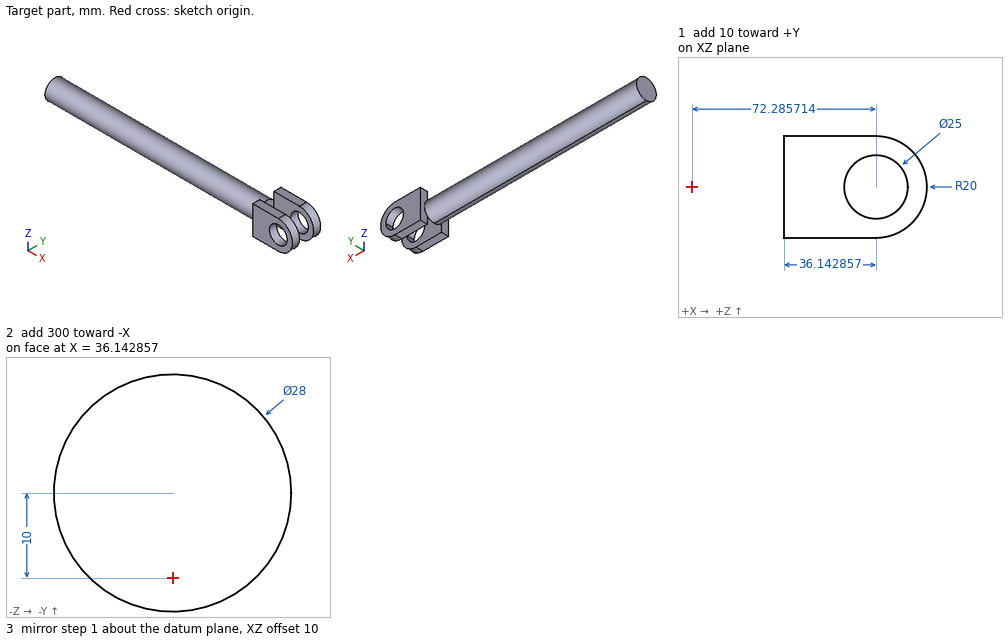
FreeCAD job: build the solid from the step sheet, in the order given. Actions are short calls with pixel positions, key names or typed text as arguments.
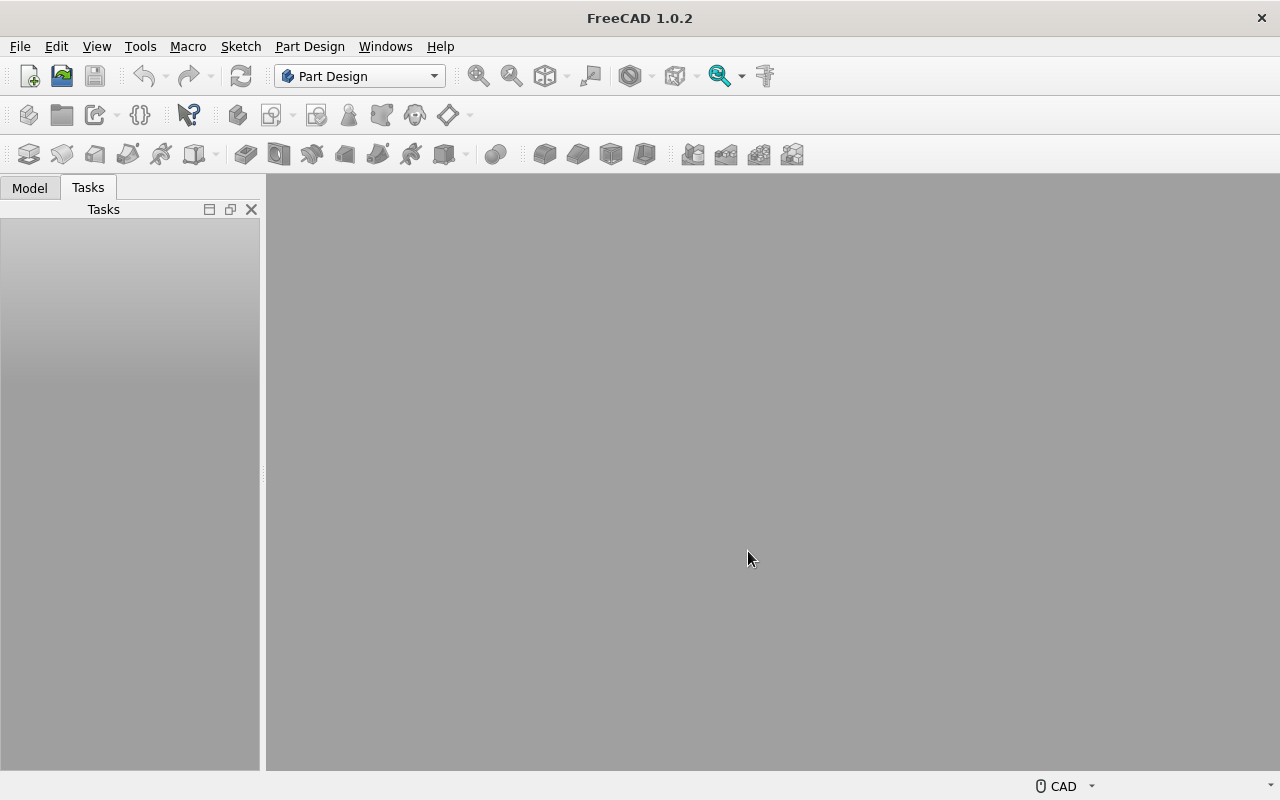
key(ctrl+n)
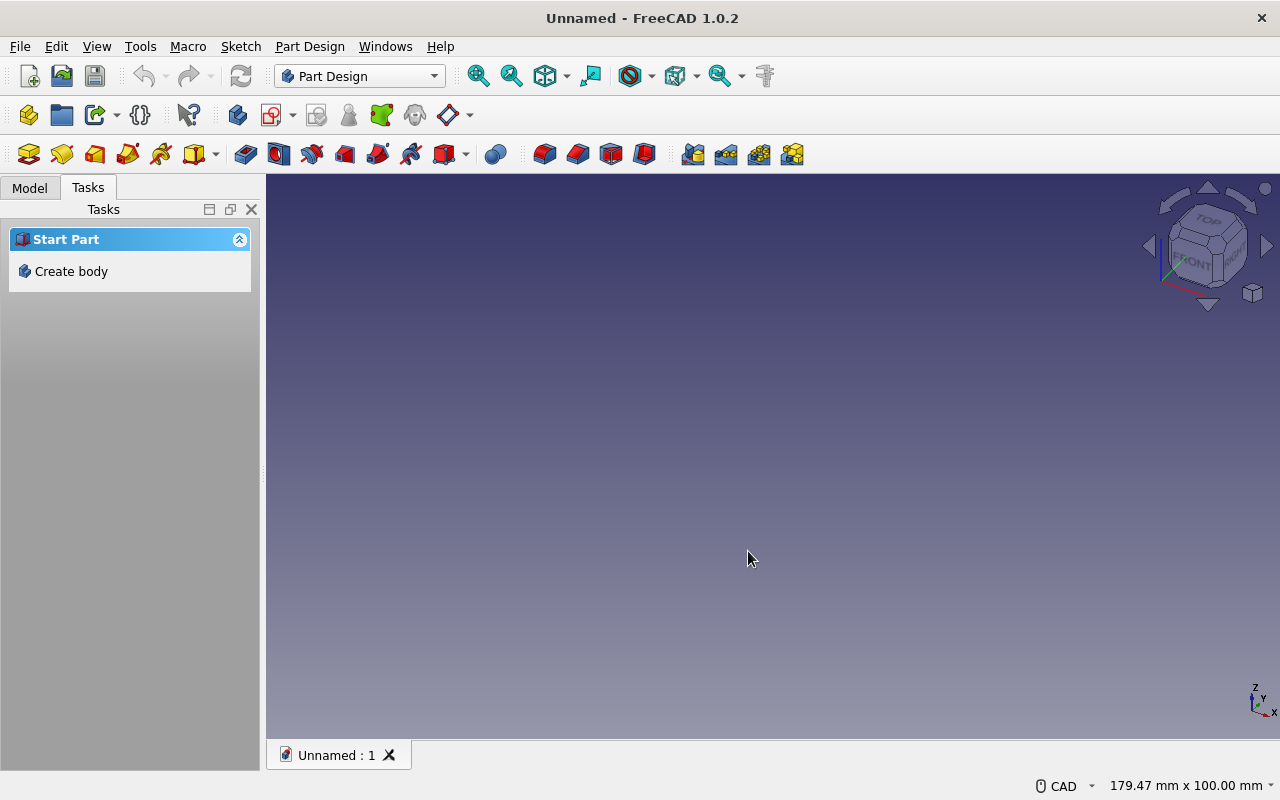
click(270, 116)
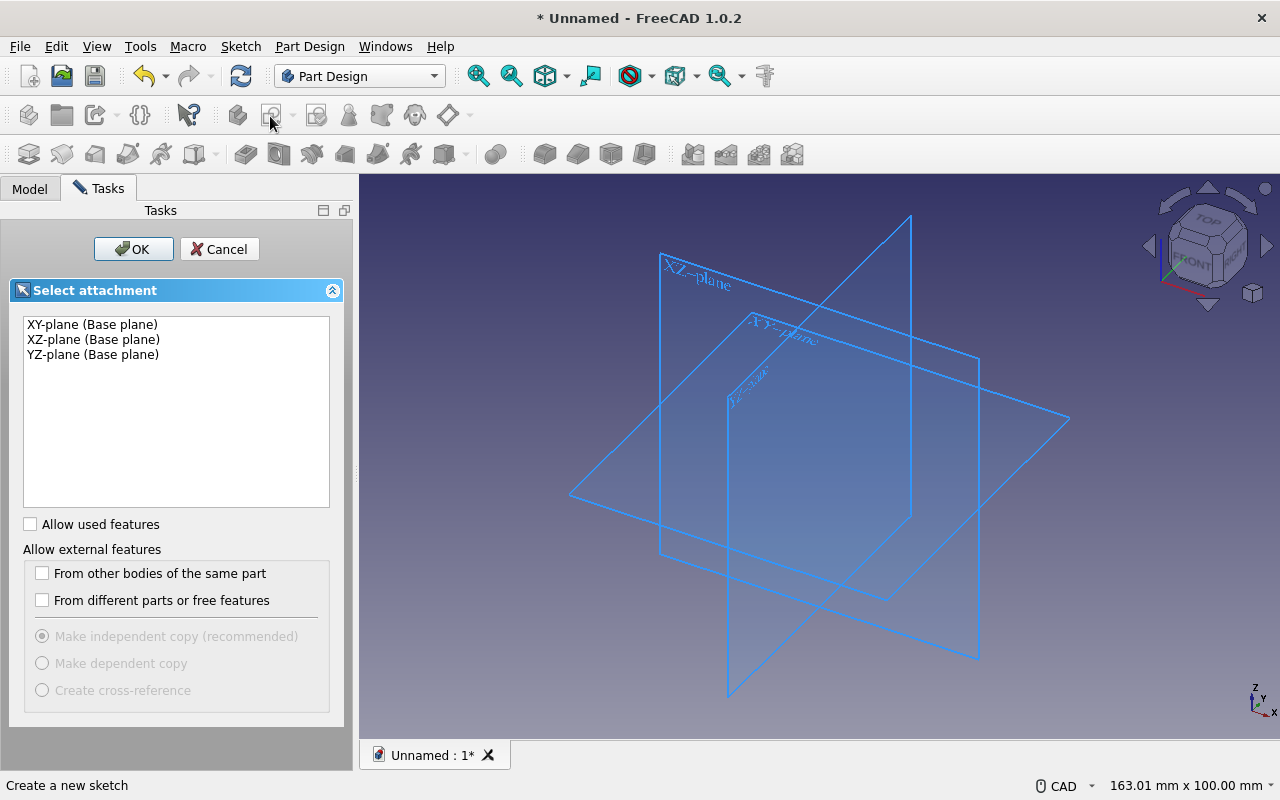
click(84, 340)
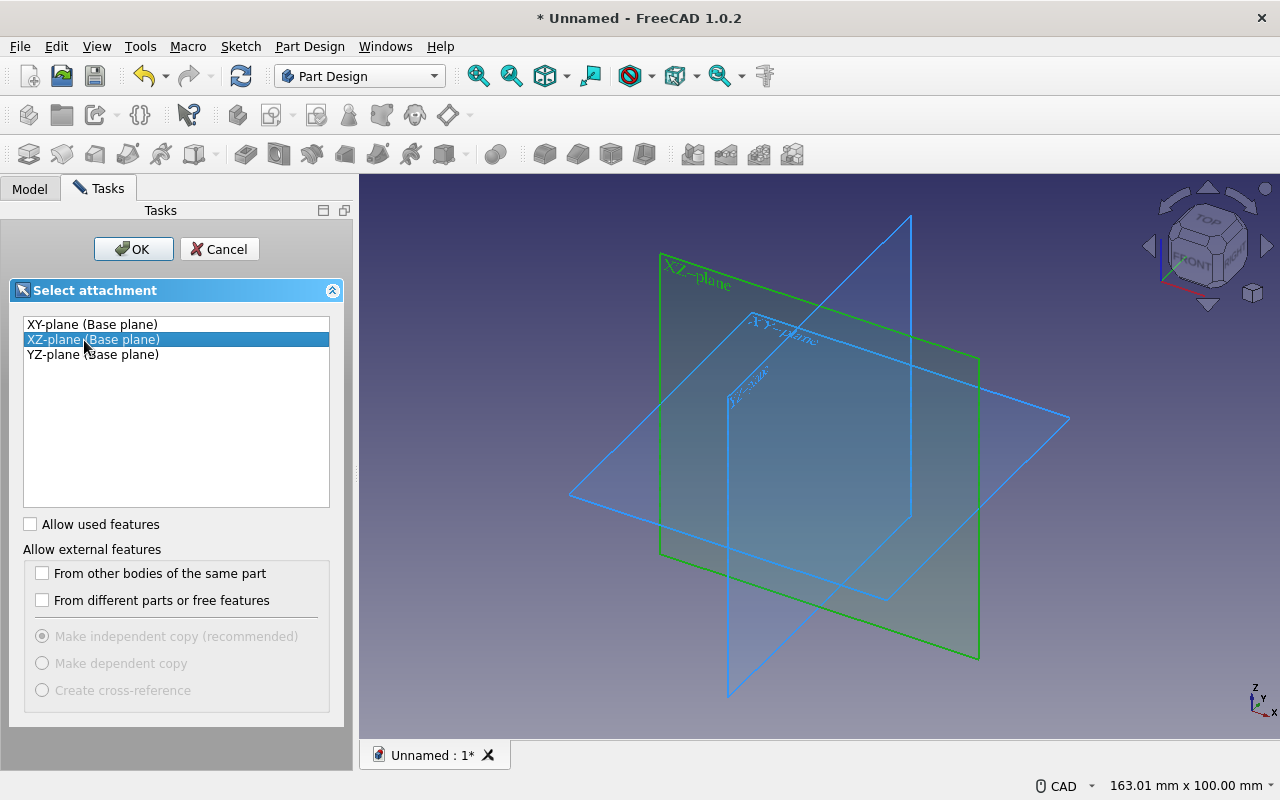
click(134, 249)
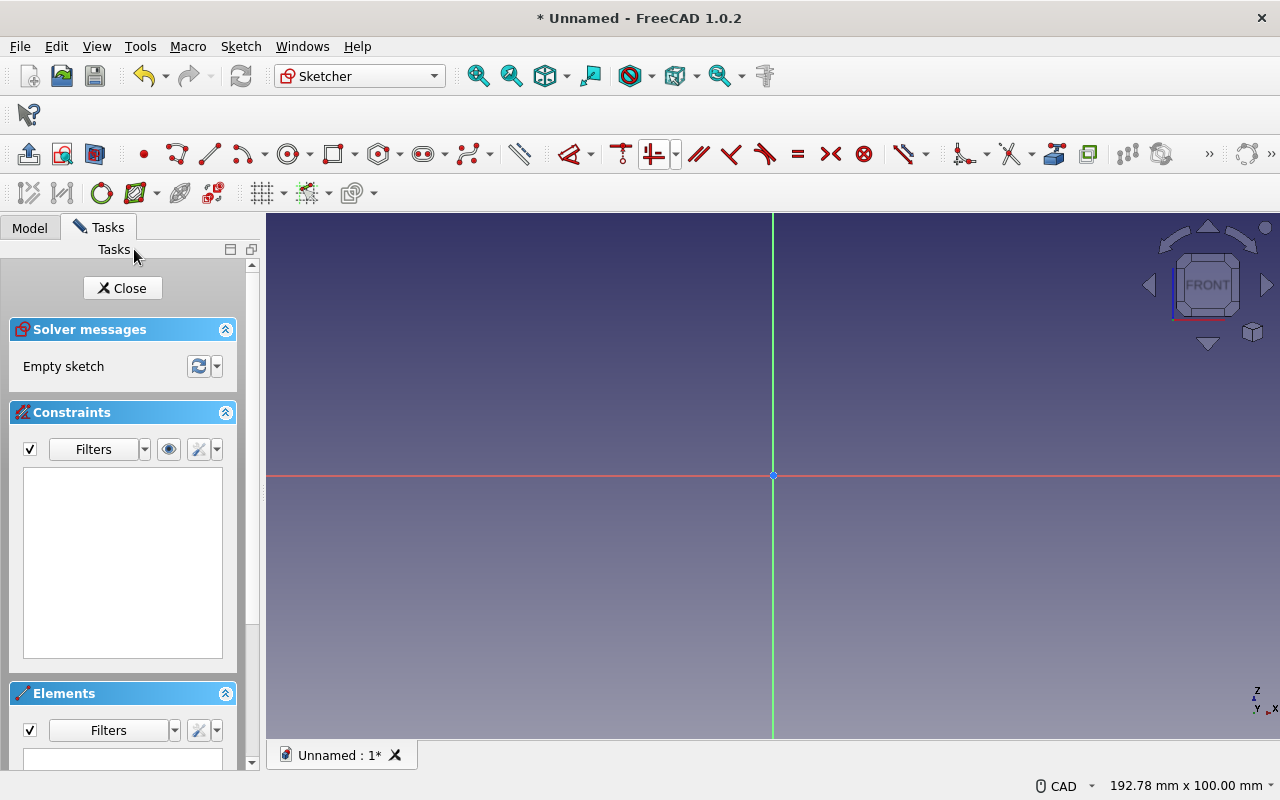
scroll(294, 476, down, 1)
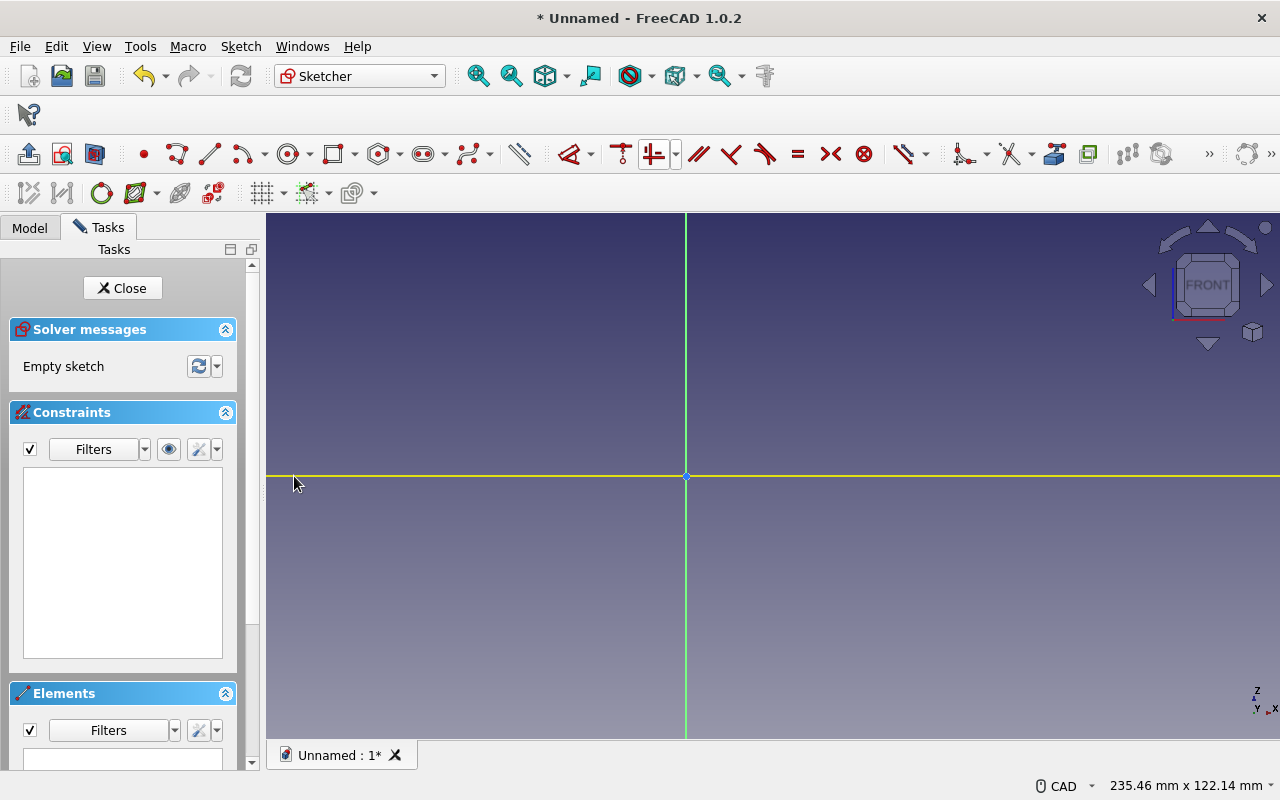
scroll(1115, 476, up, 2)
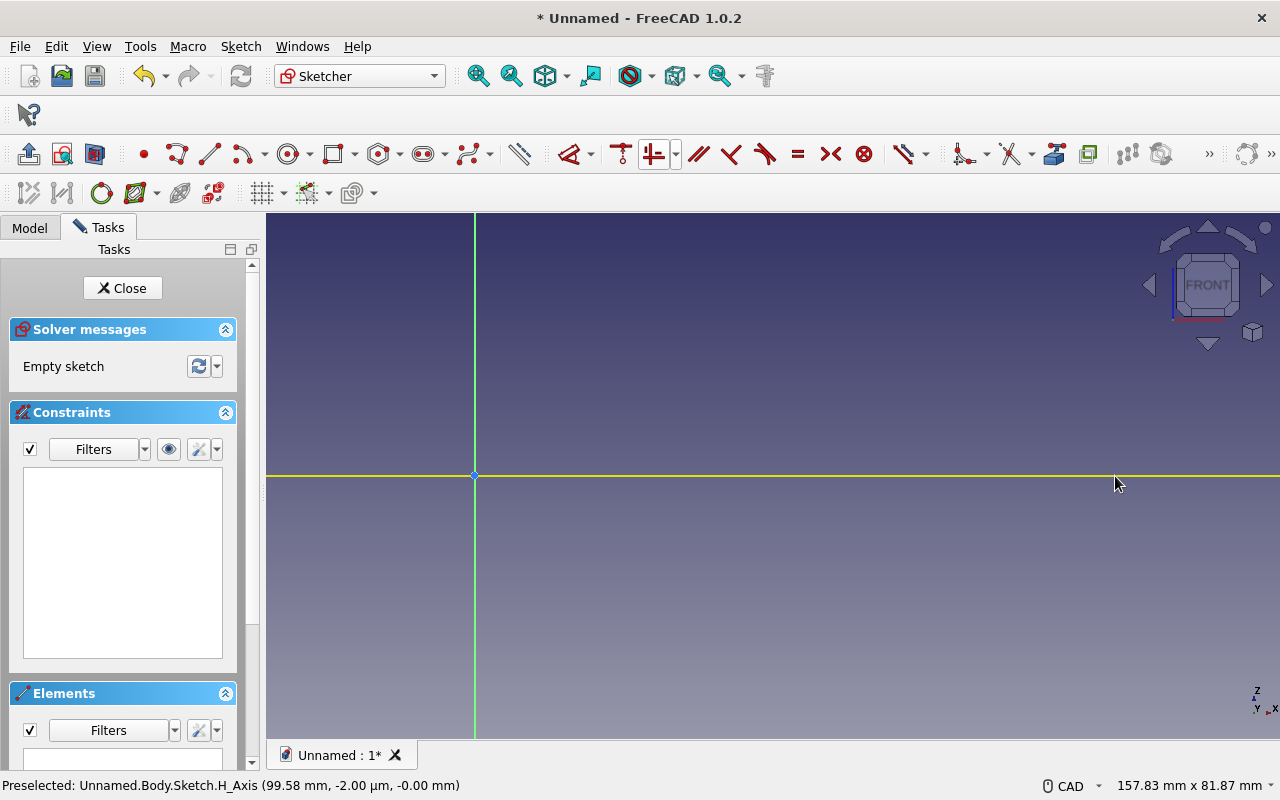
key(g)
key(m)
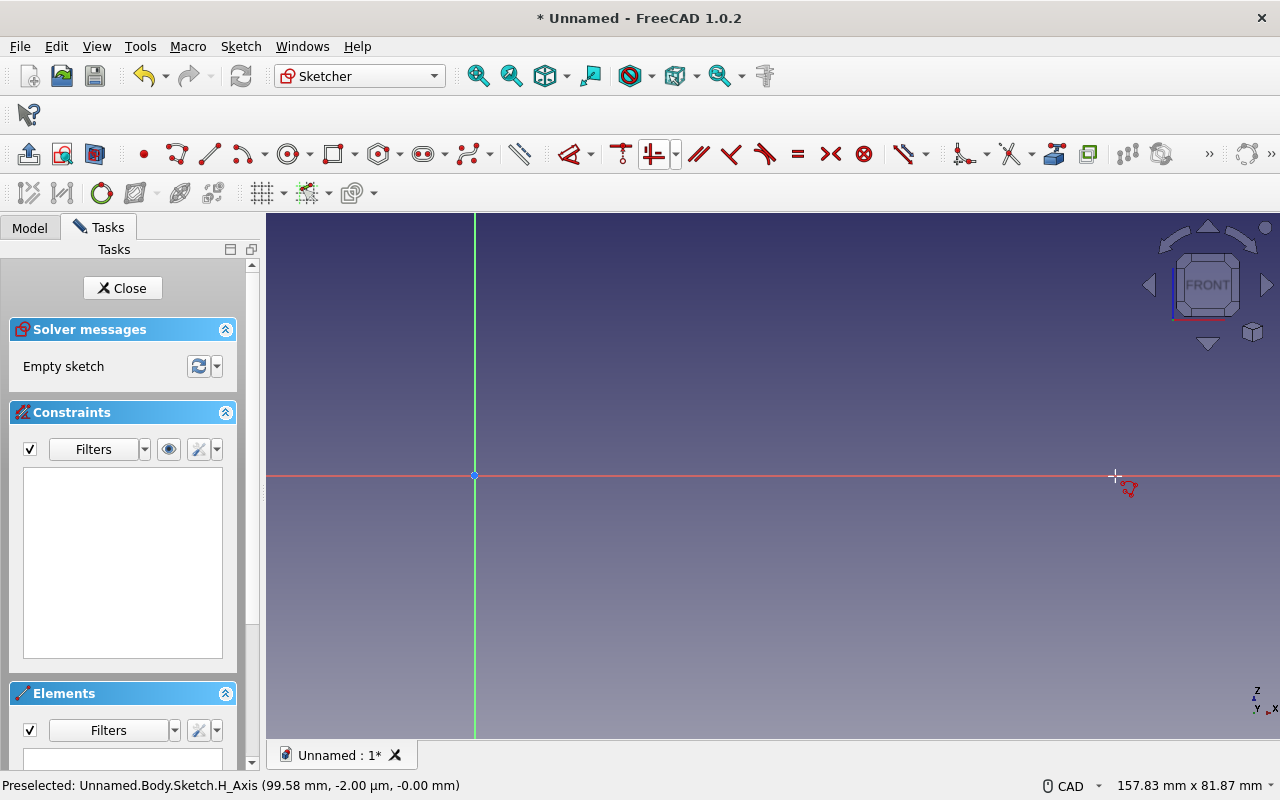
click(939, 604)
click(707, 604)
click(707, 347)
click(939, 347)
right_click(939, 347)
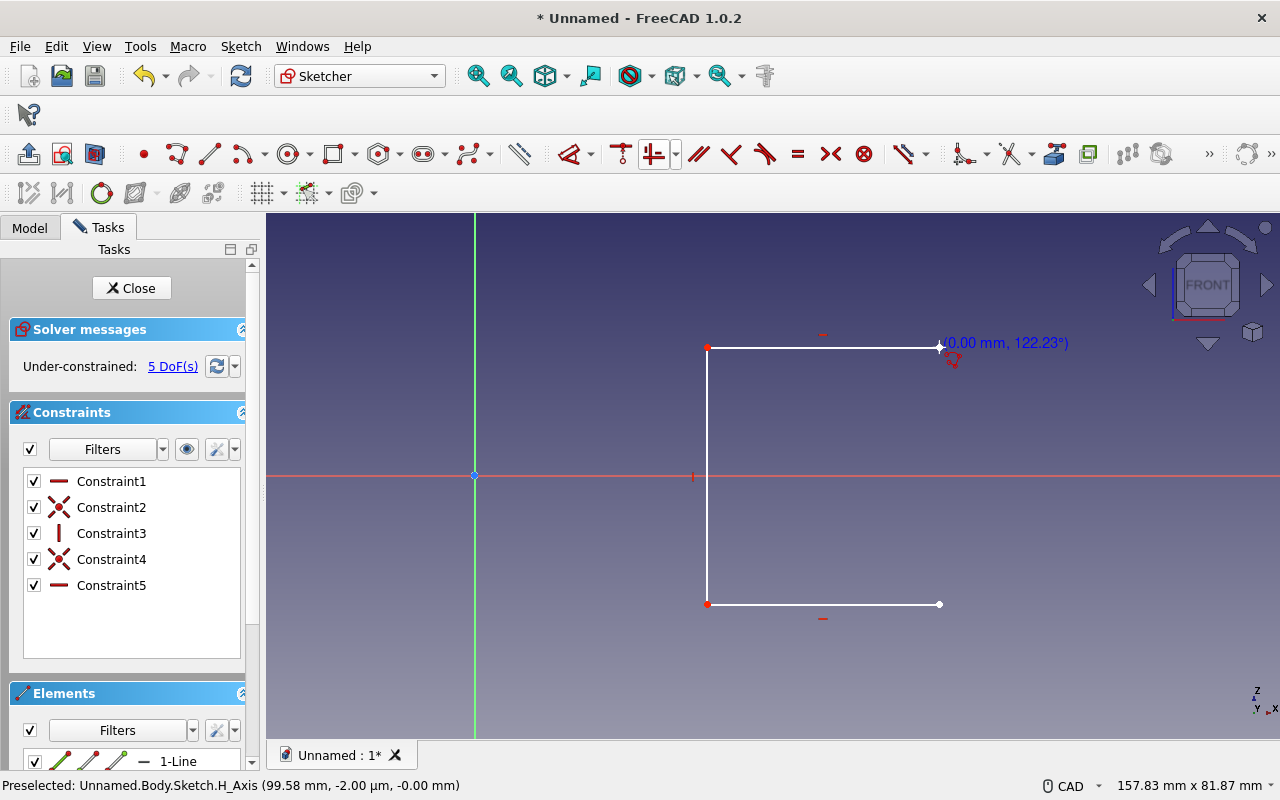
key(g)
key(3)
key(a)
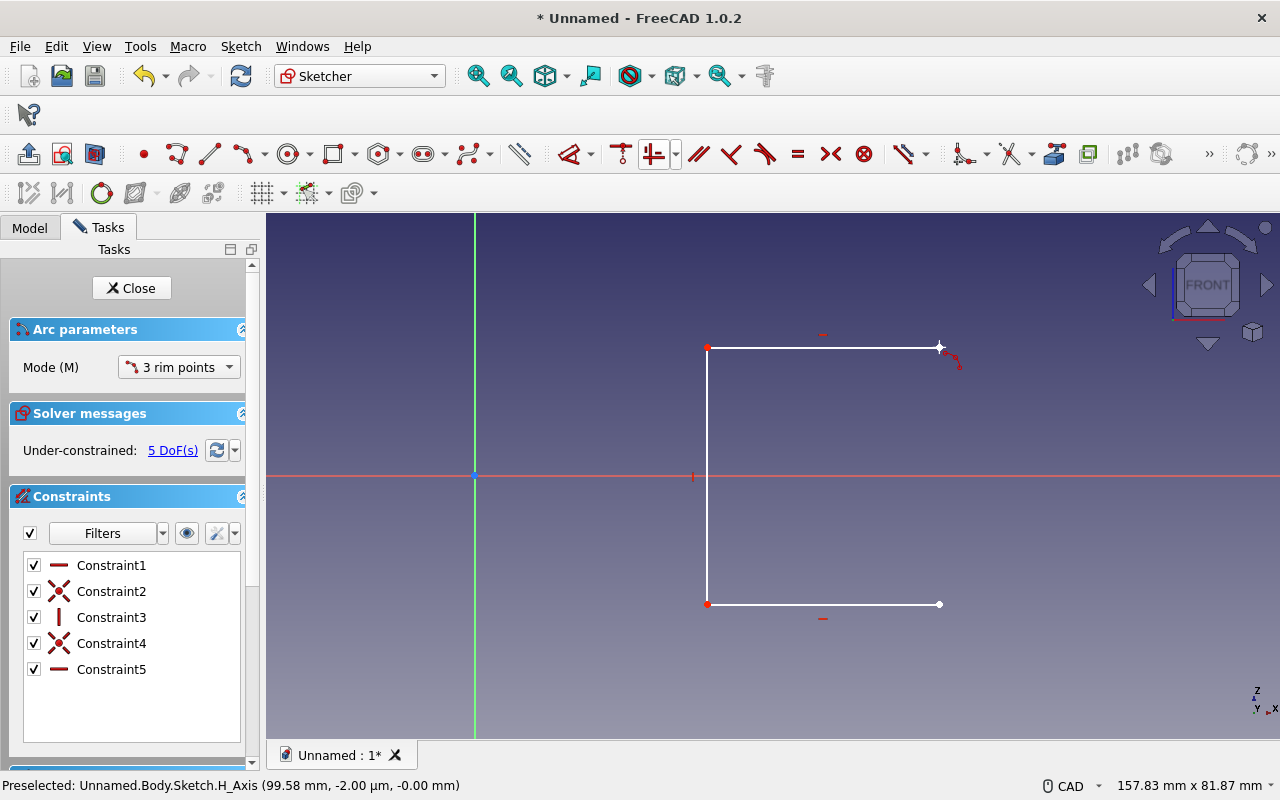
click(939, 348)
click(939, 605)
click(1061, 516)